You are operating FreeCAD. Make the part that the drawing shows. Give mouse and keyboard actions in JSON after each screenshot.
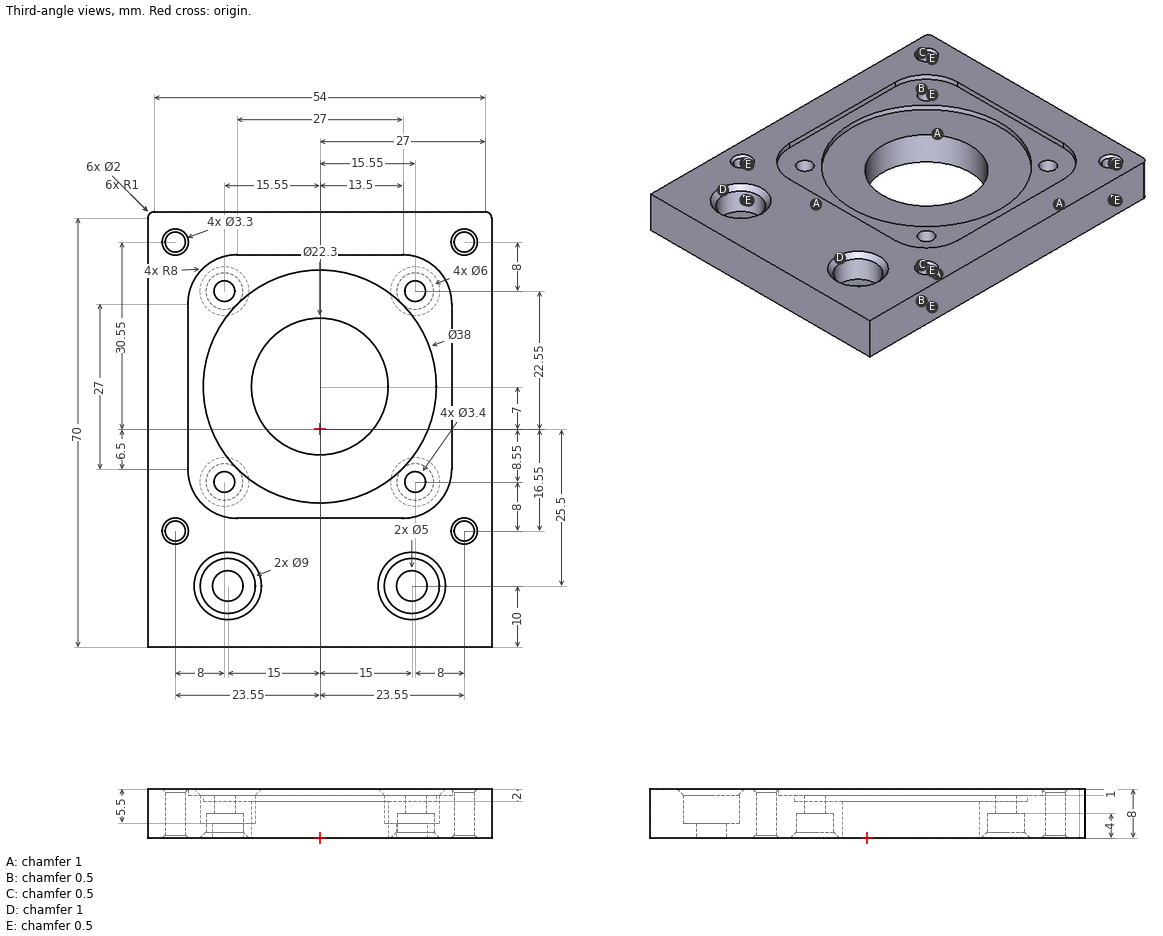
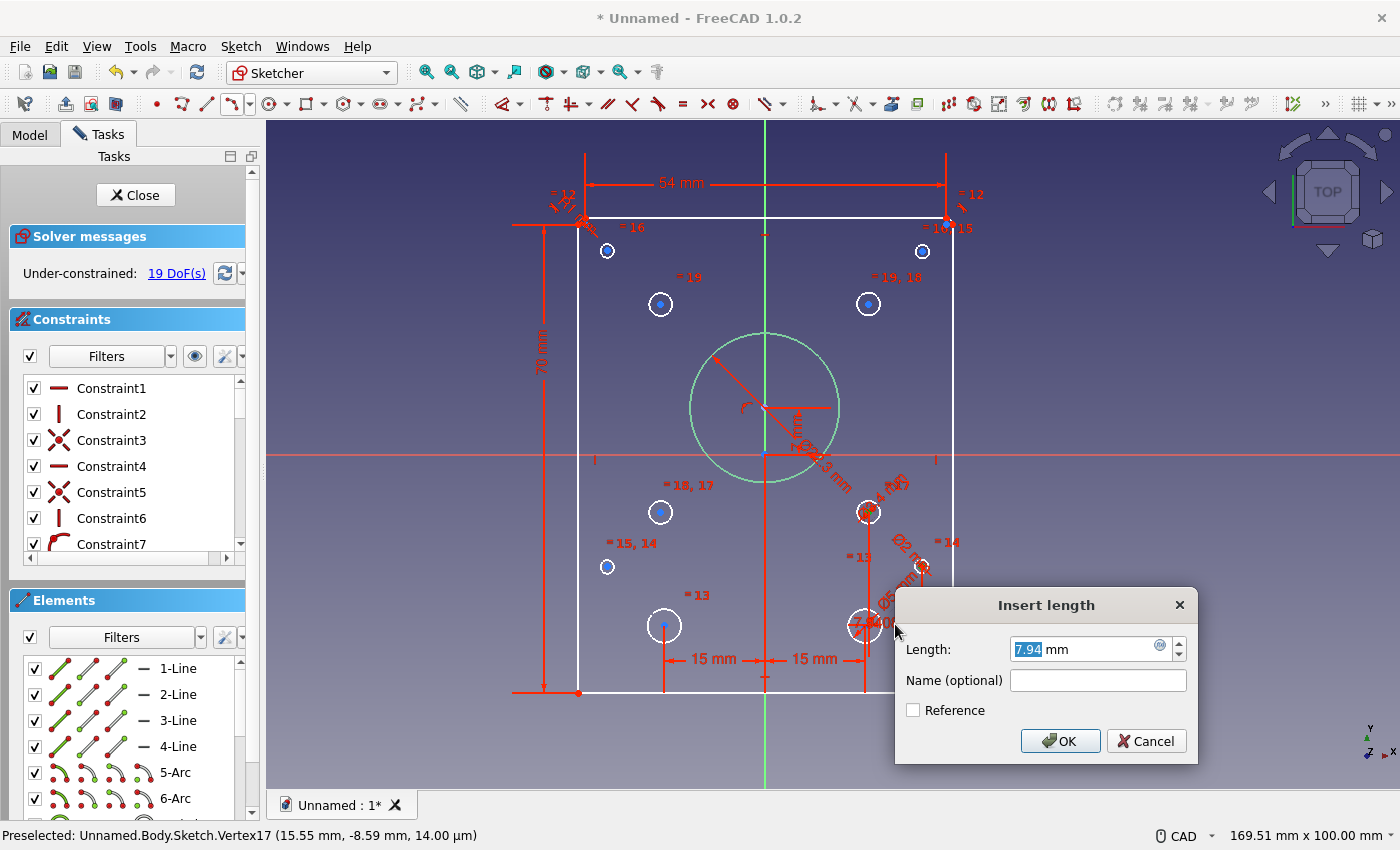
{"action": "type", "text": "8"}
{"action": "key", "text": "Return"}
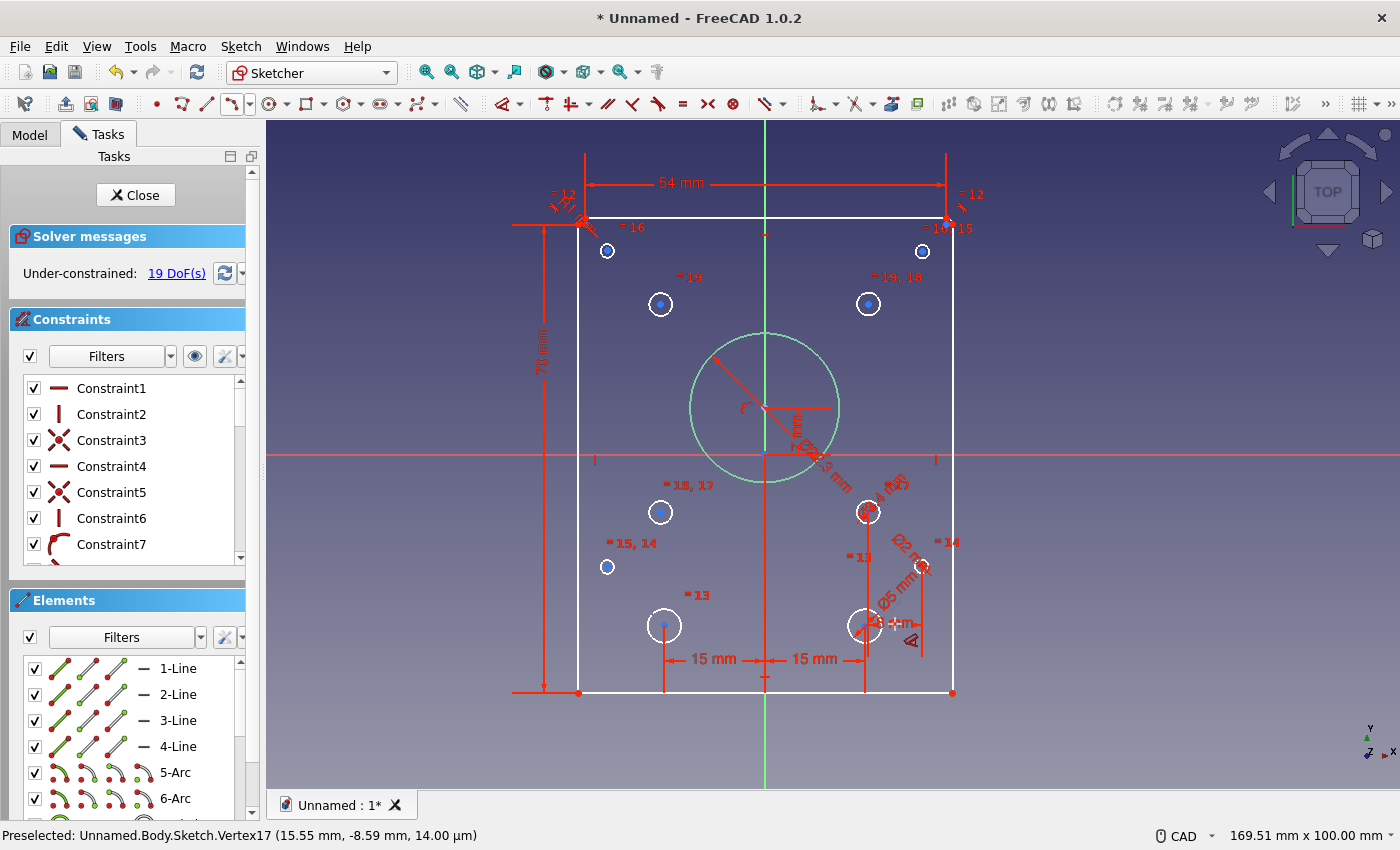
{"action": "left_click", "coordinate": [922, 566]}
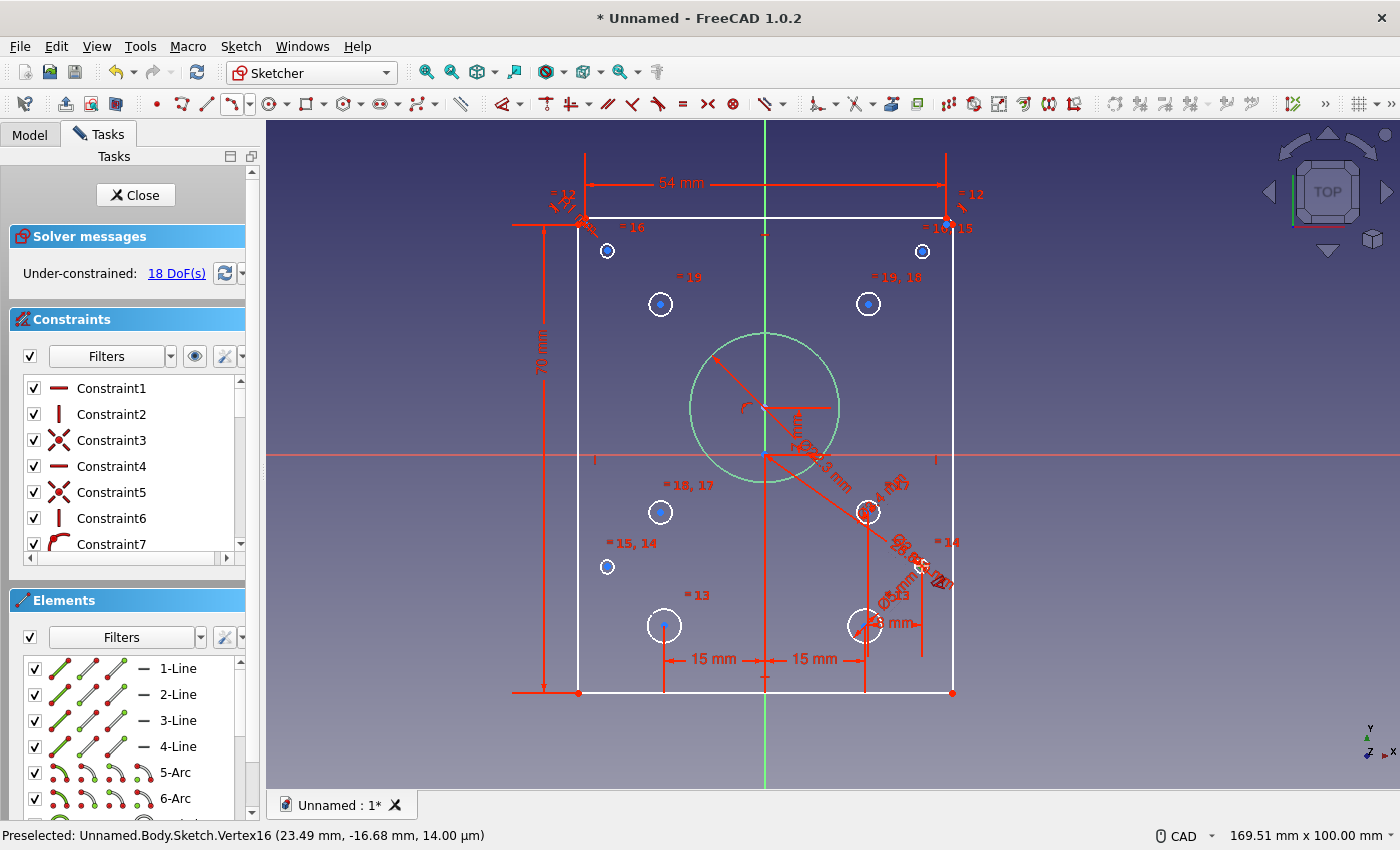
{"action": "left_click", "coordinate": [868, 512]}
{"action": "left_click", "coordinate": [834, 539]}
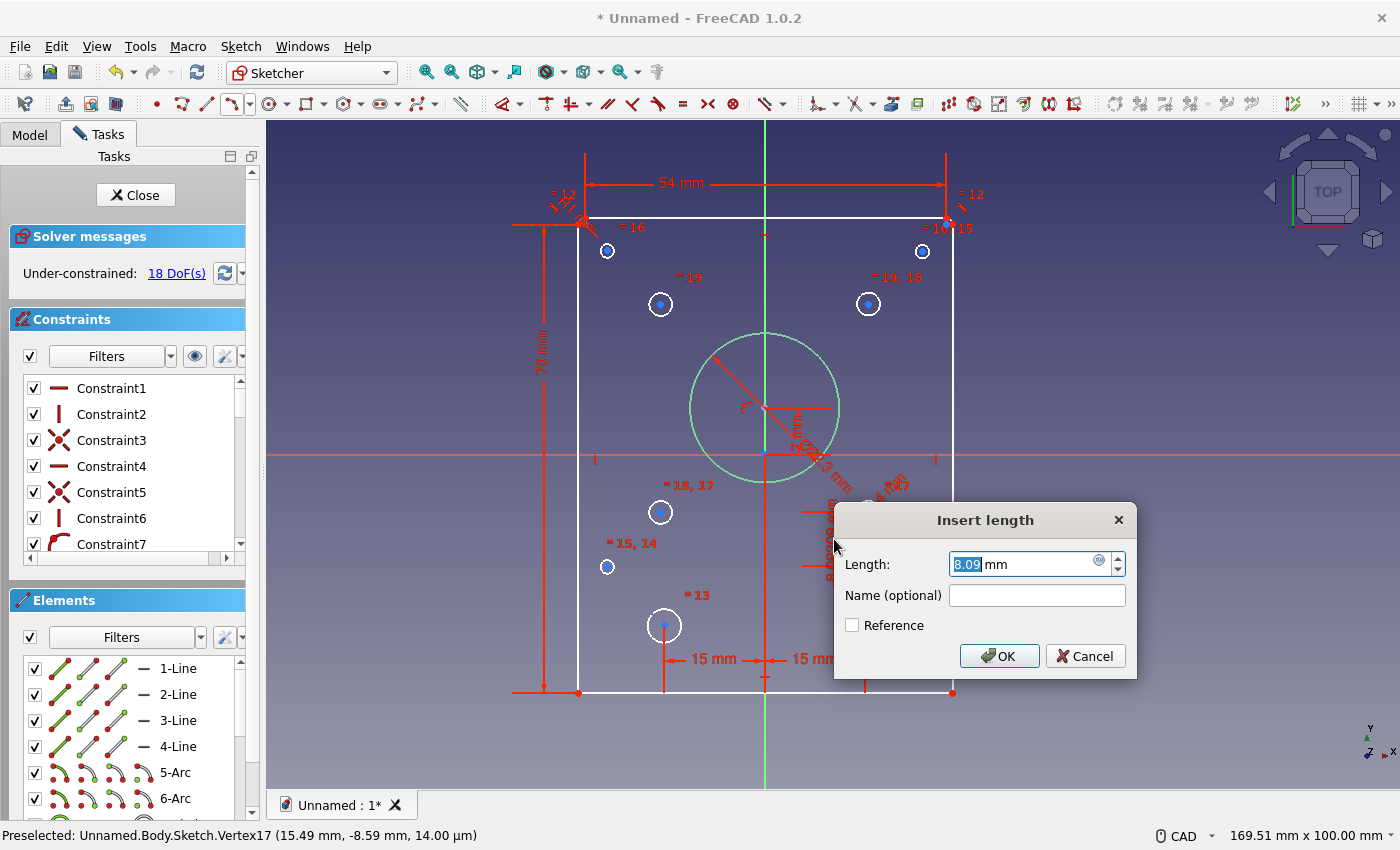
{"action": "type", "text": "8"}
{"action": "key", "text": "Return"}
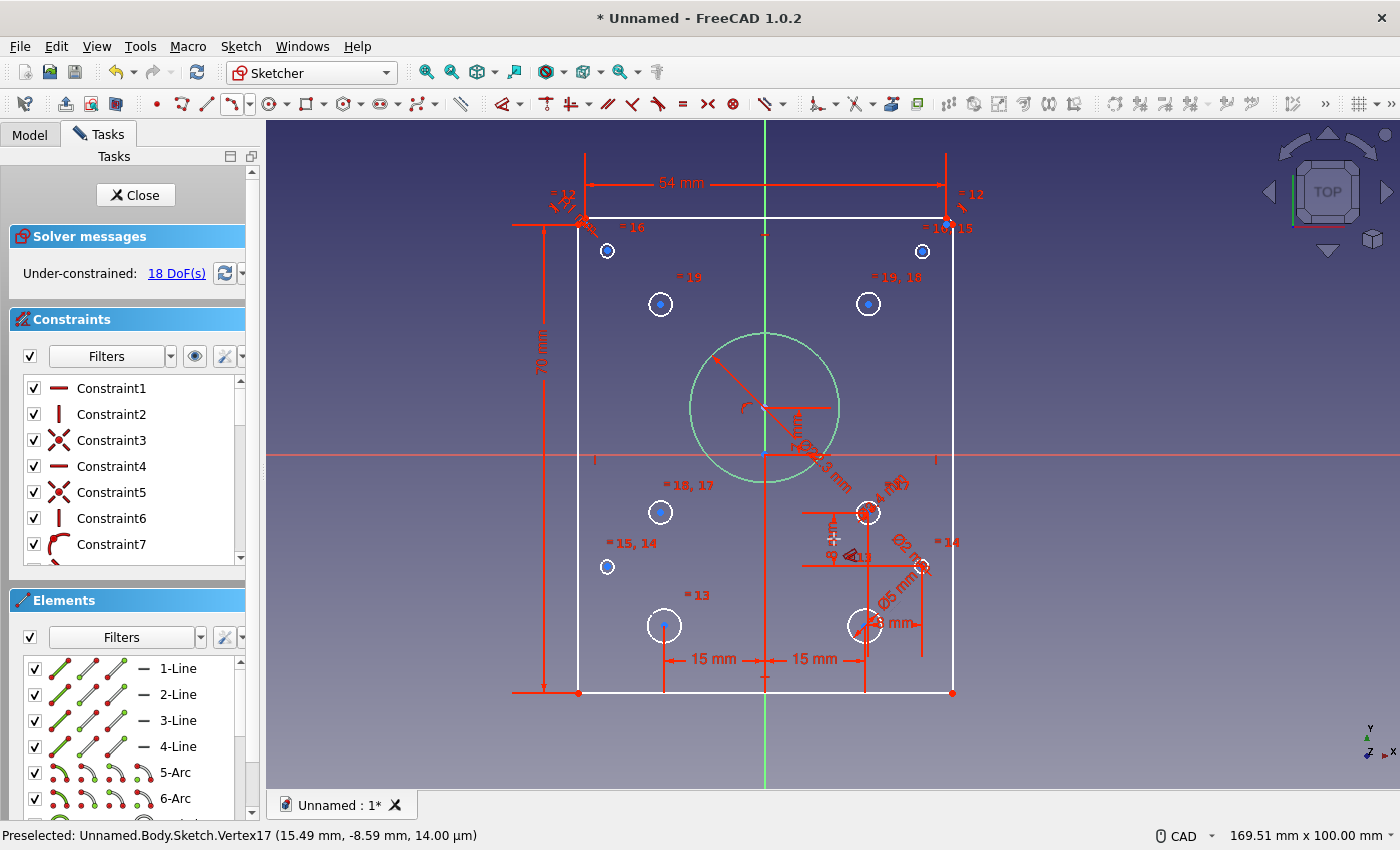
{"action": "left_click", "coordinate": [868, 513]}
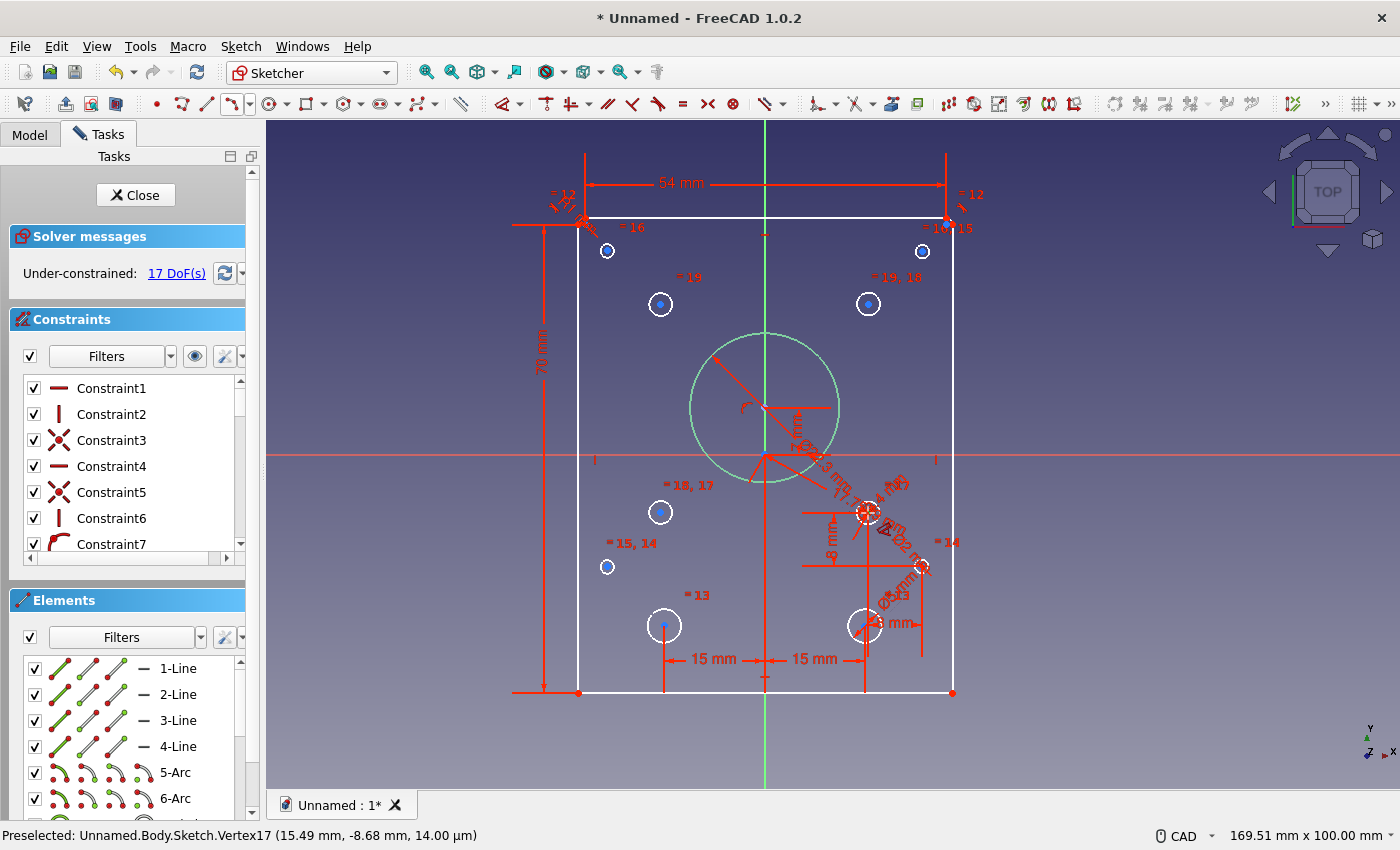
{"action": "left_click", "coordinate": [607, 567]}
{"action": "left_click", "coordinate": [549, 540]}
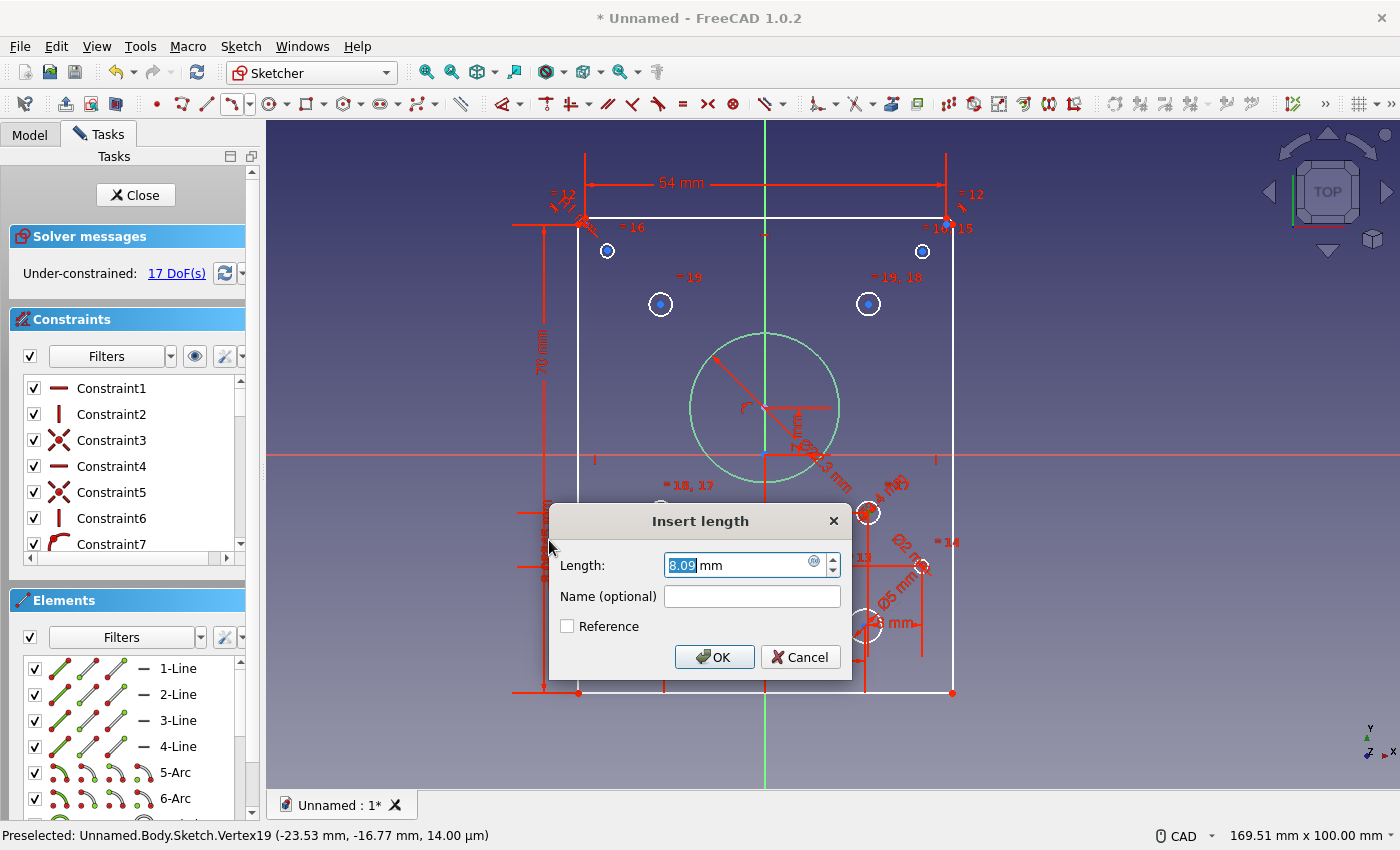
{"action": "type", "text": "8"}
{"action": "key", "text": "Return"}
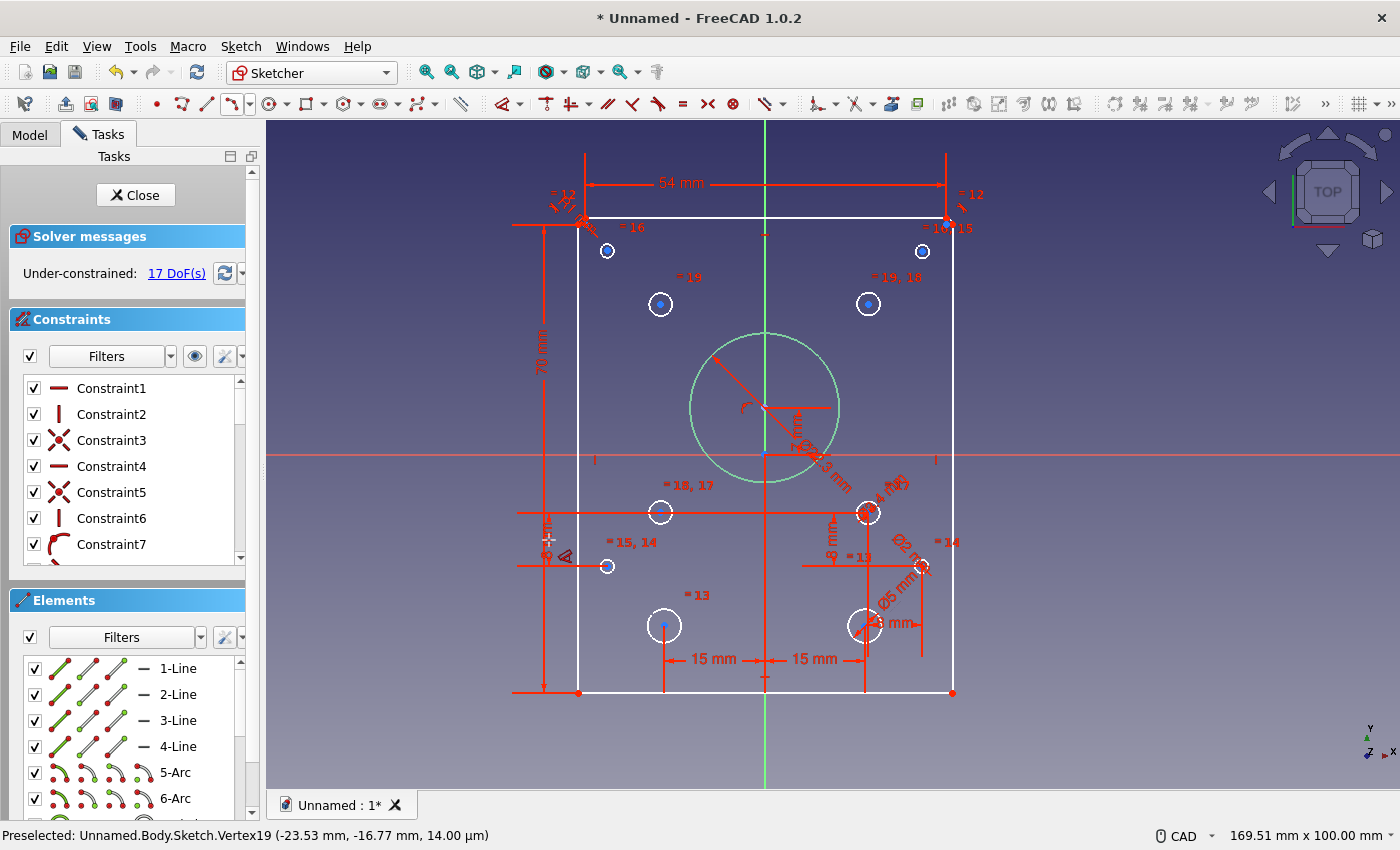
{"action": "left_click", "coordinate": [607, 566]}